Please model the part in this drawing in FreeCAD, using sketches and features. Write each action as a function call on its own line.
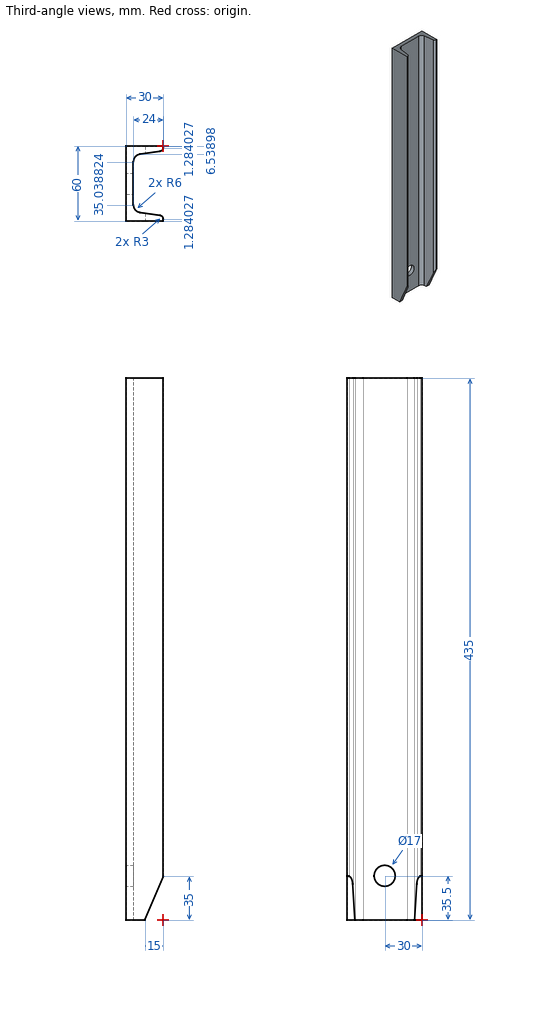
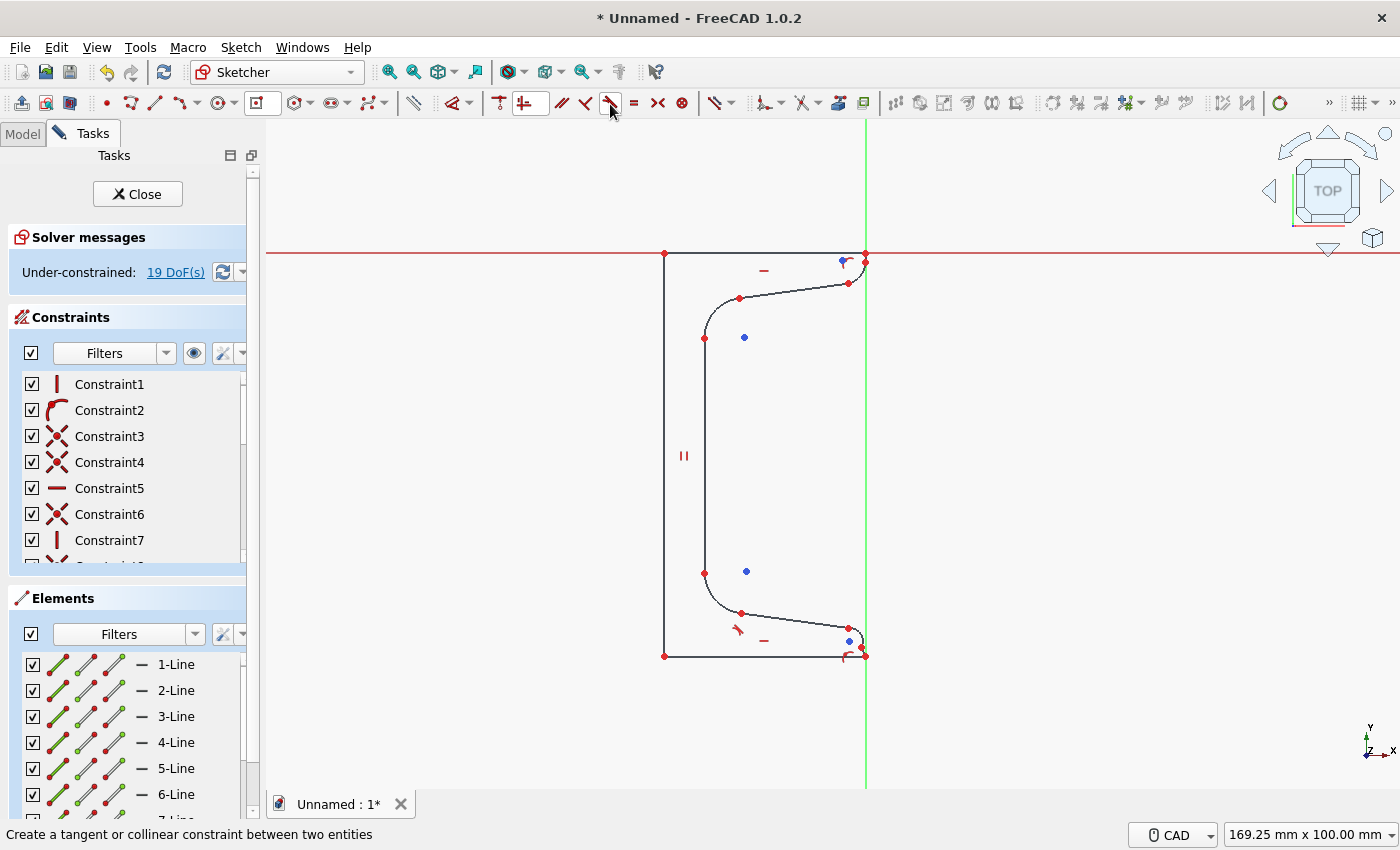
click(816, 624)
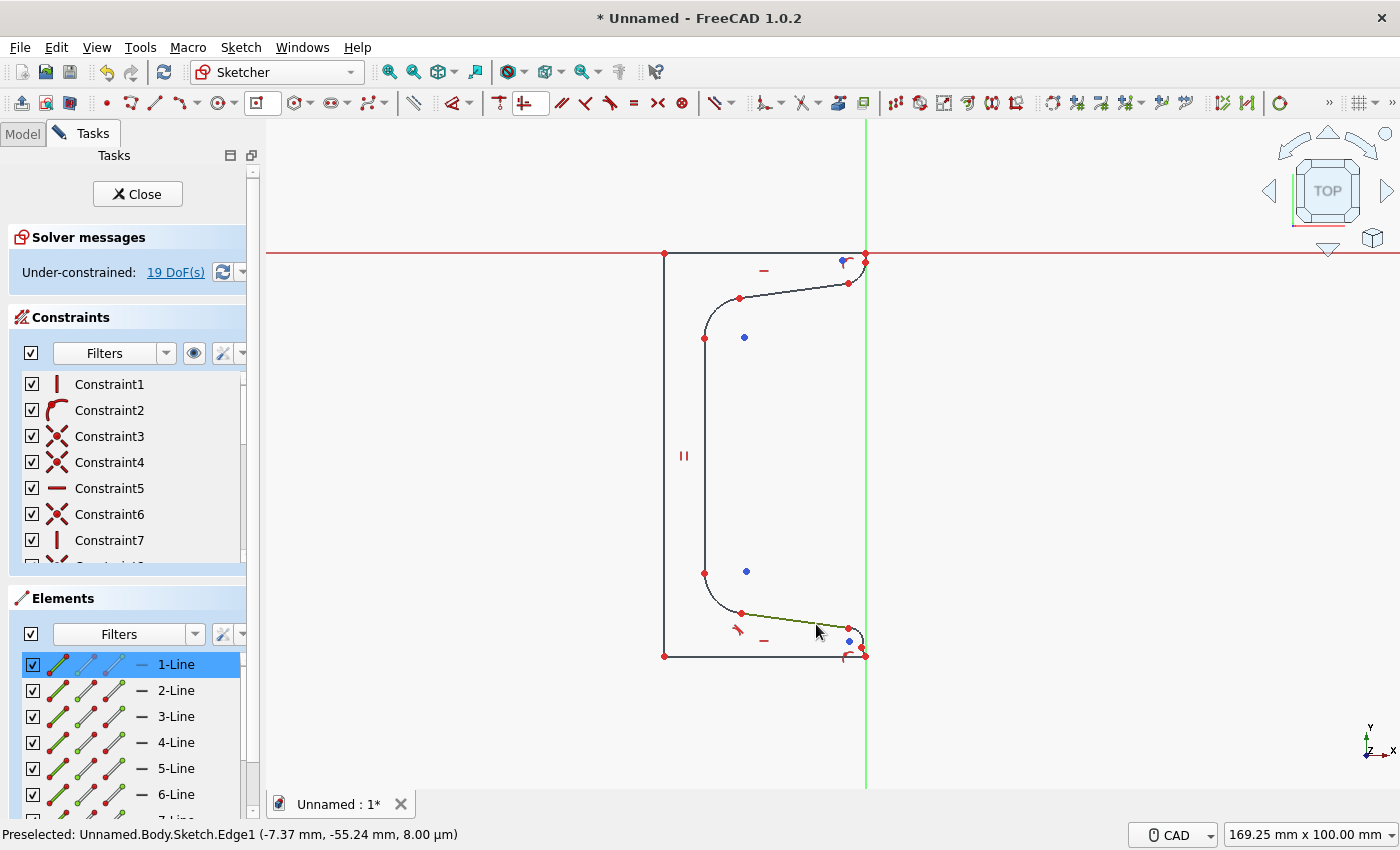
scroll(857, 630, up, 3)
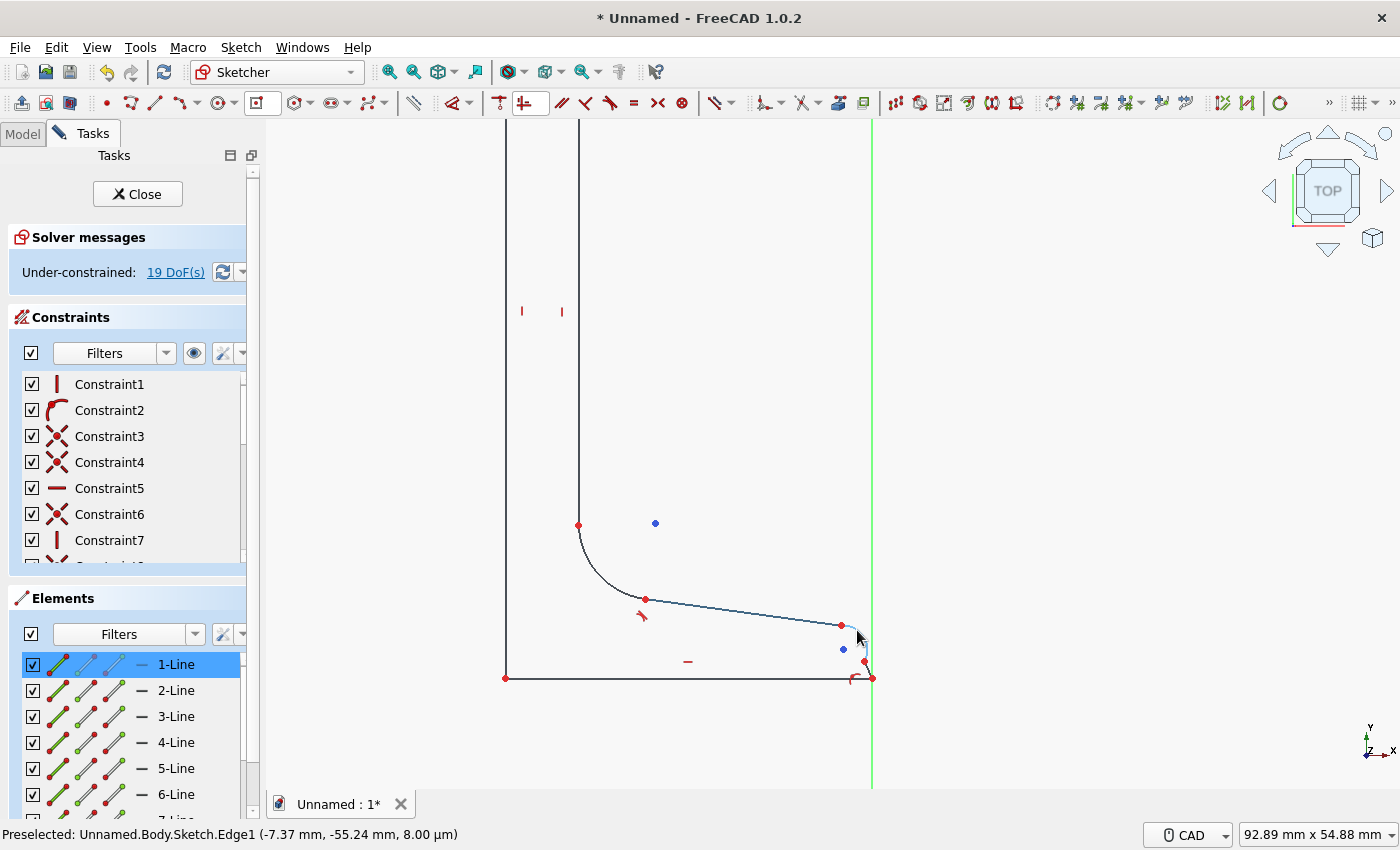
click(856, 629)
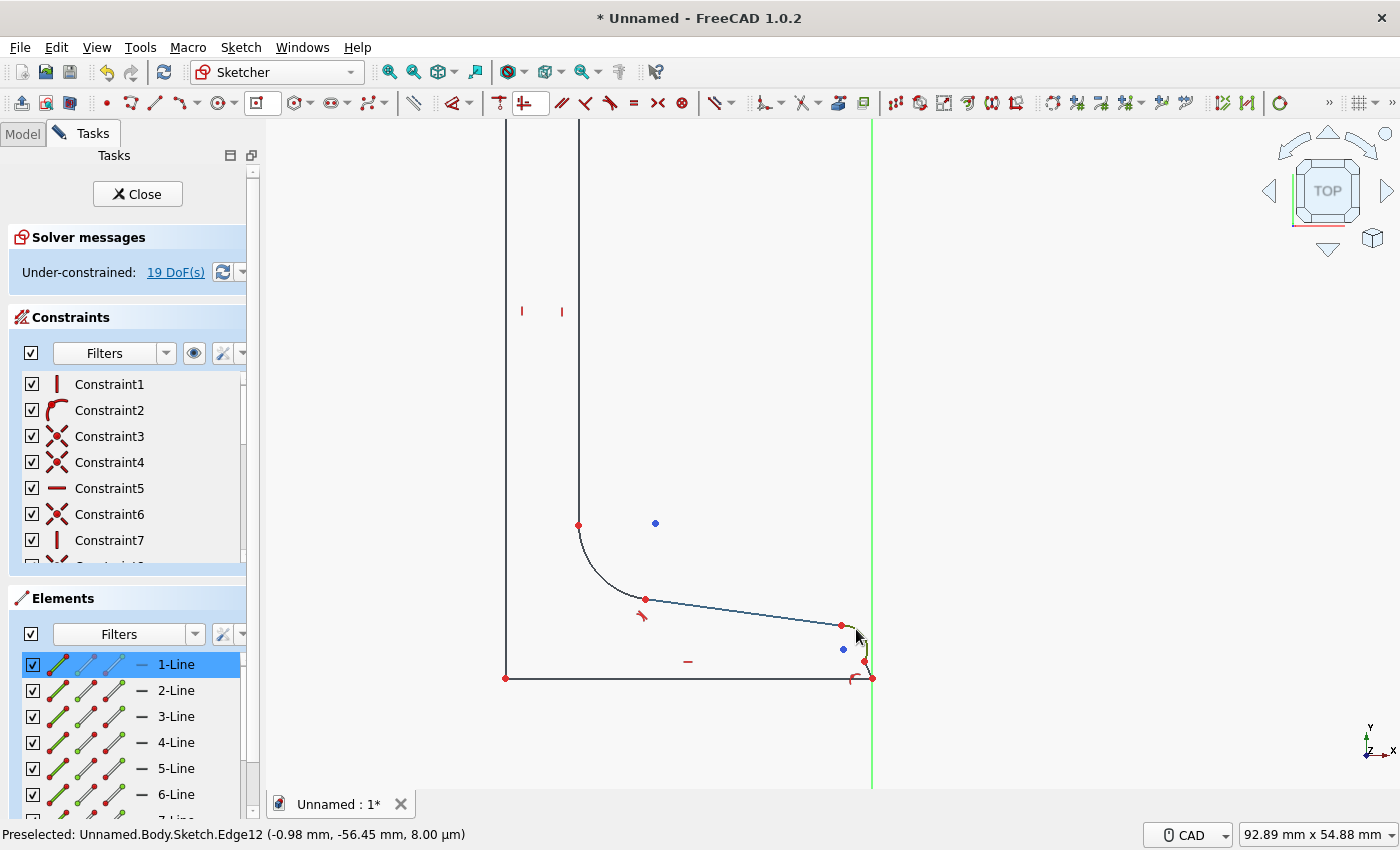
click(610, 104)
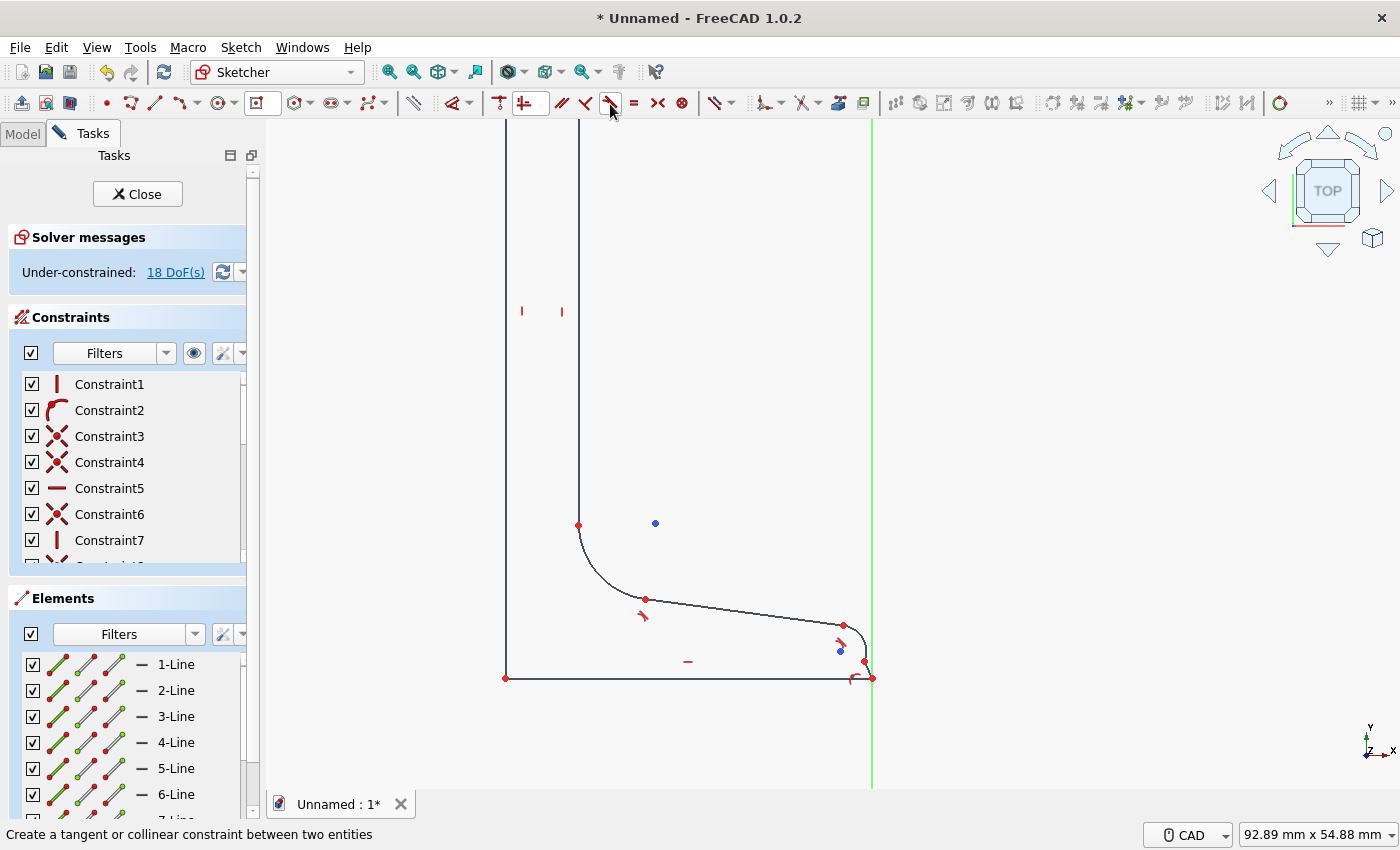
click(579, 397)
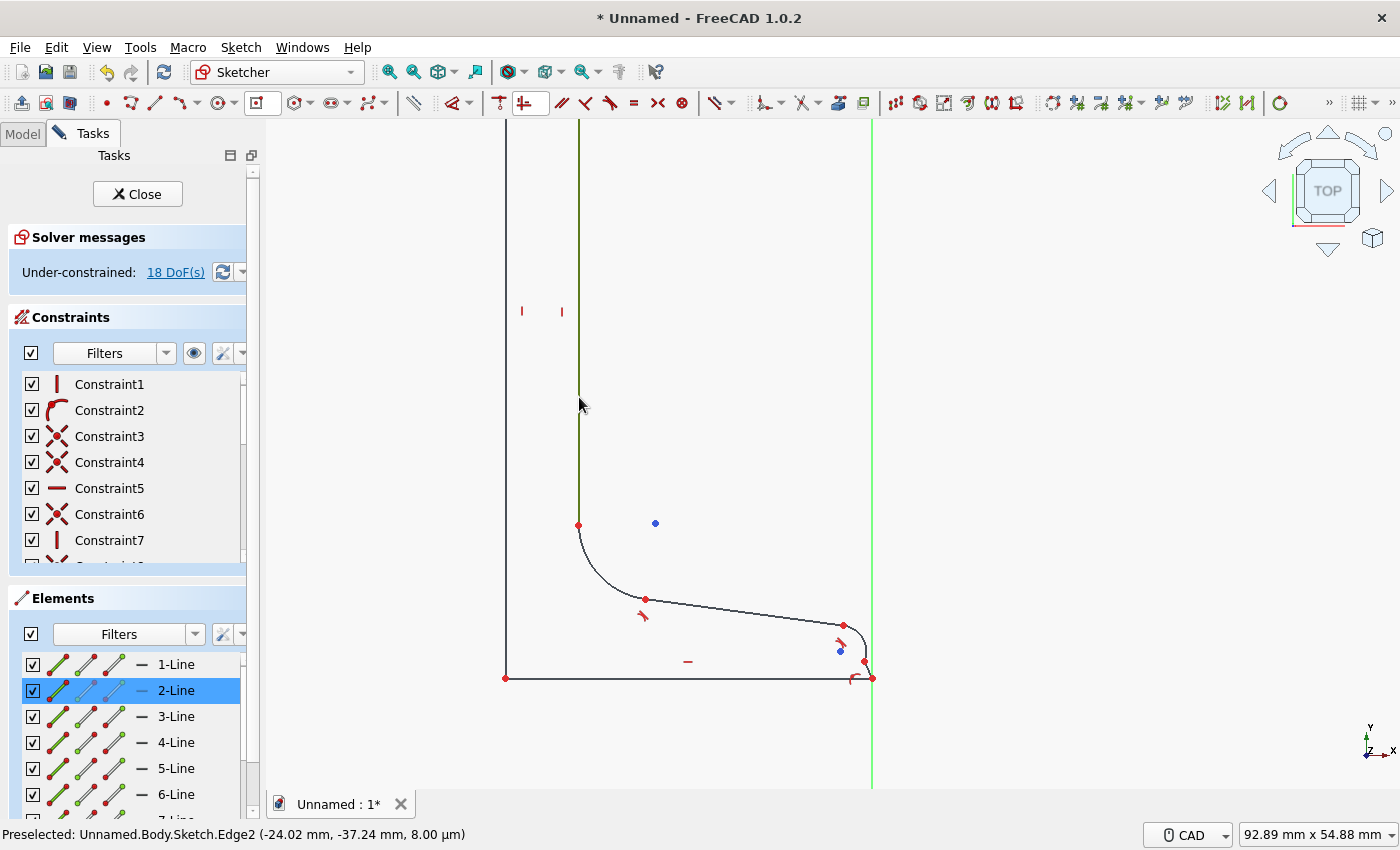
click(587, 557)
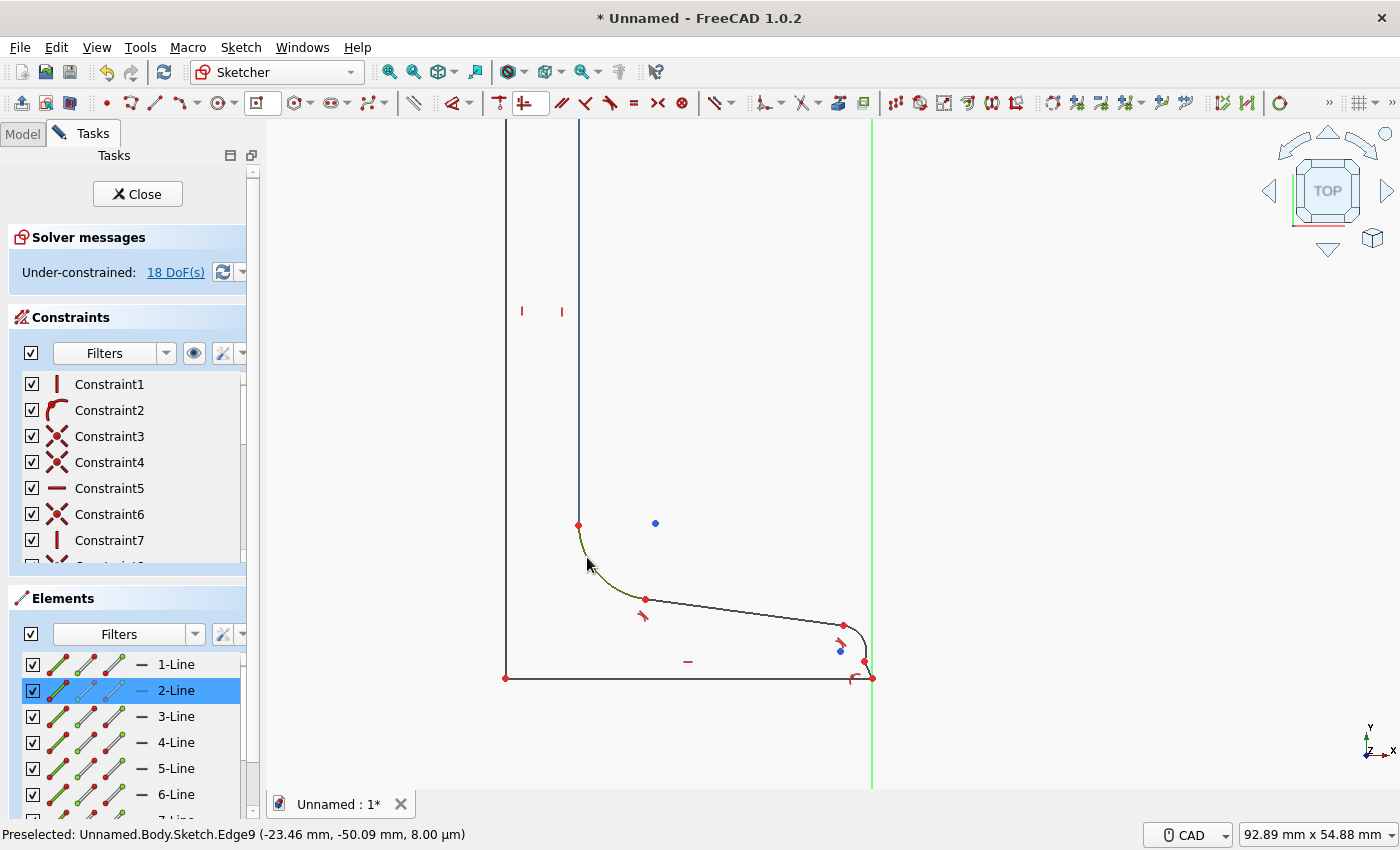
click(610, 104)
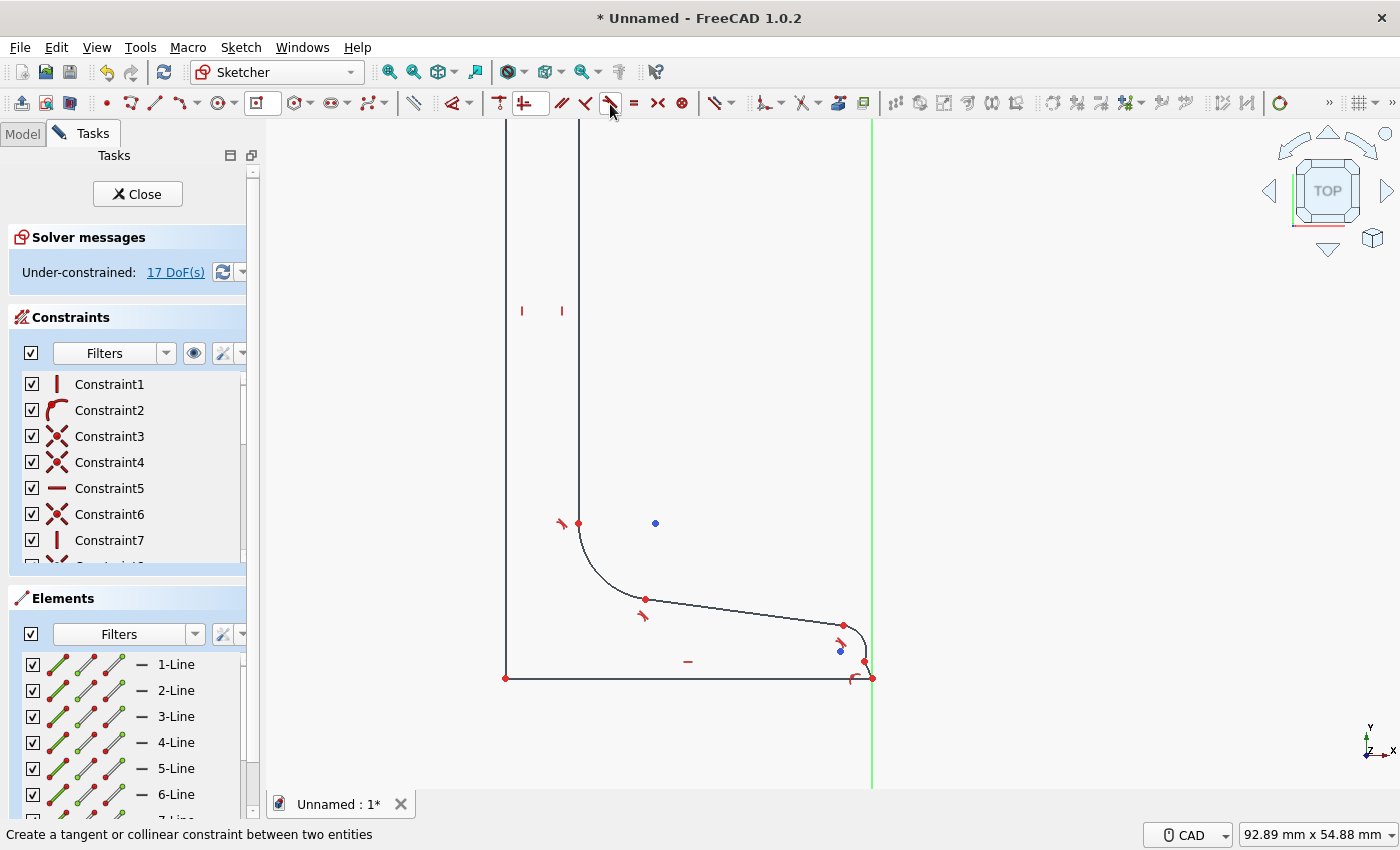
click(579, 396)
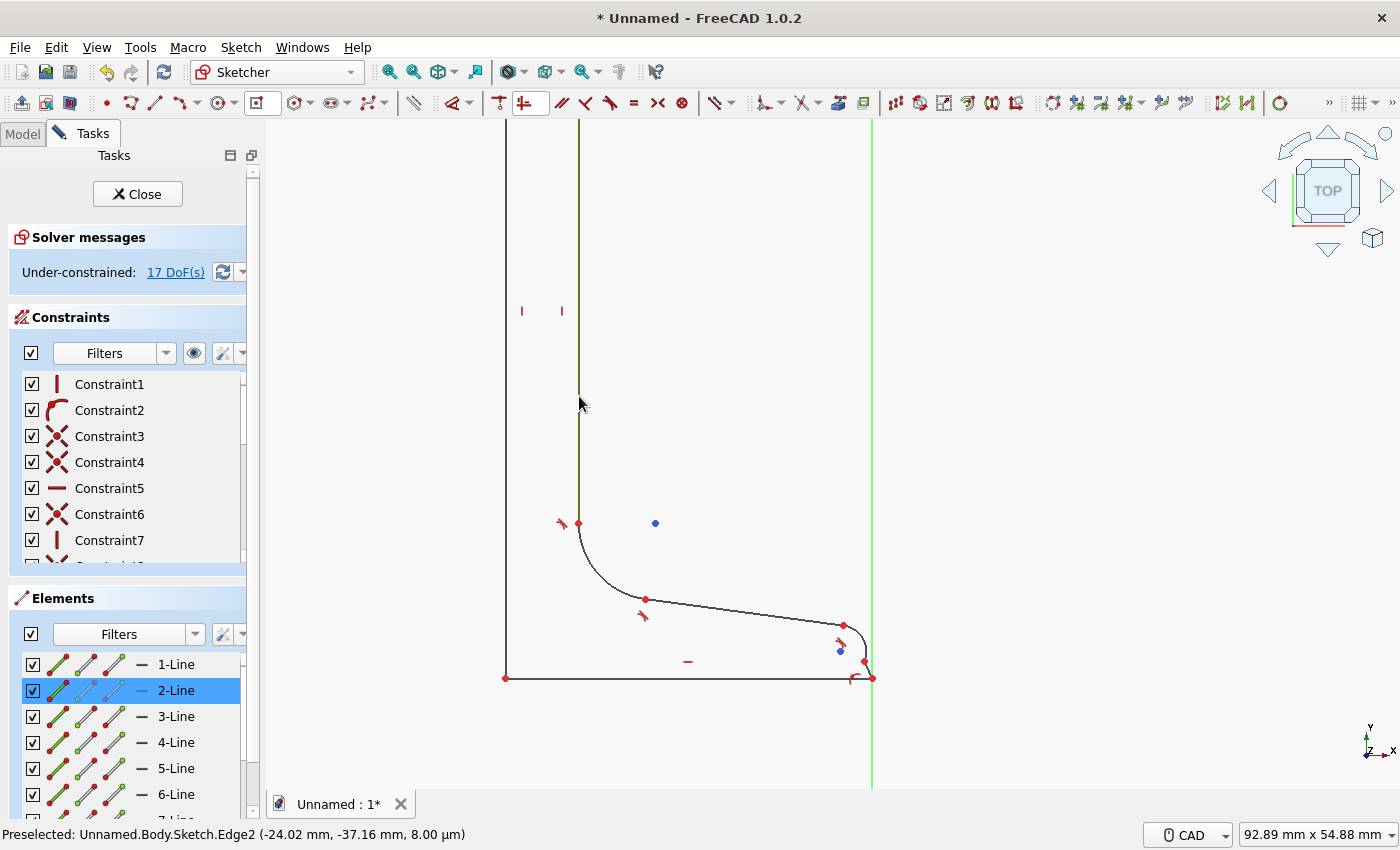
scroll(856, 630, down, 3)